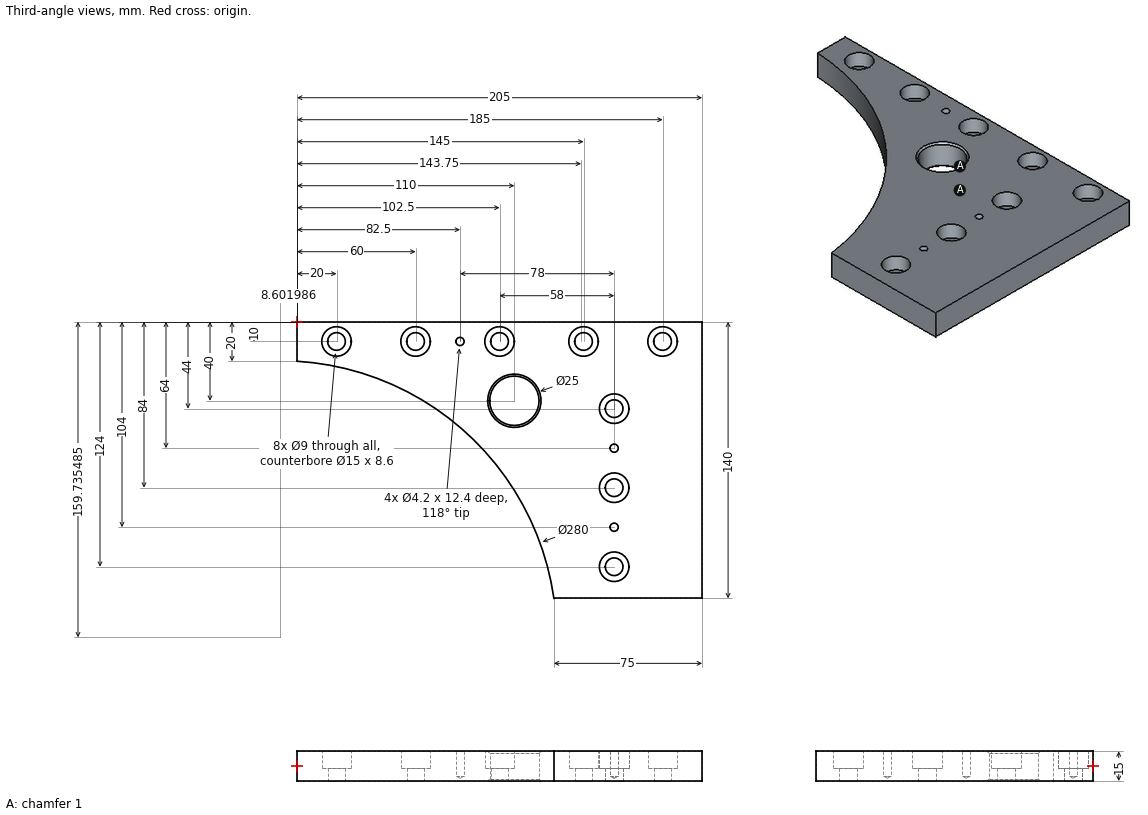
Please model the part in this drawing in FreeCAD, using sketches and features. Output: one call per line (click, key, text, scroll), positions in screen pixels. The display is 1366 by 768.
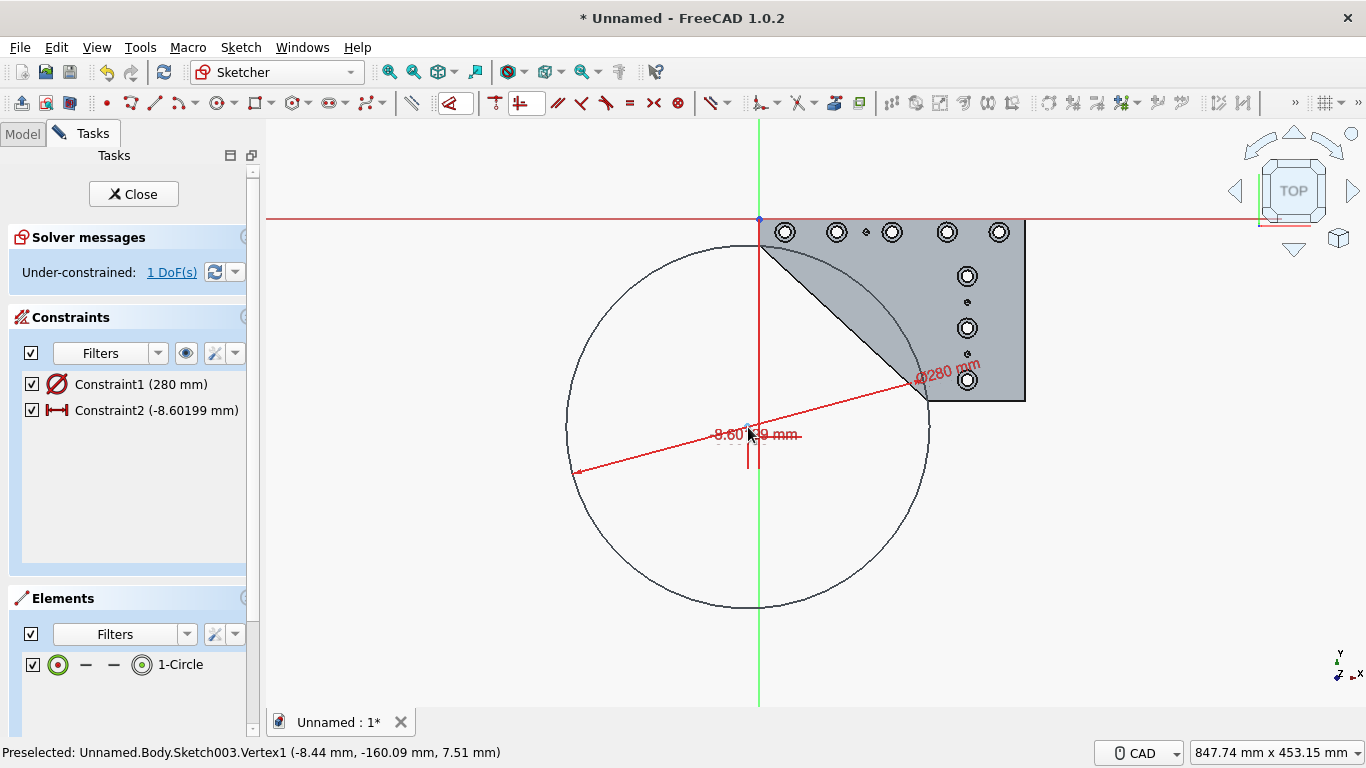
click(748, 427)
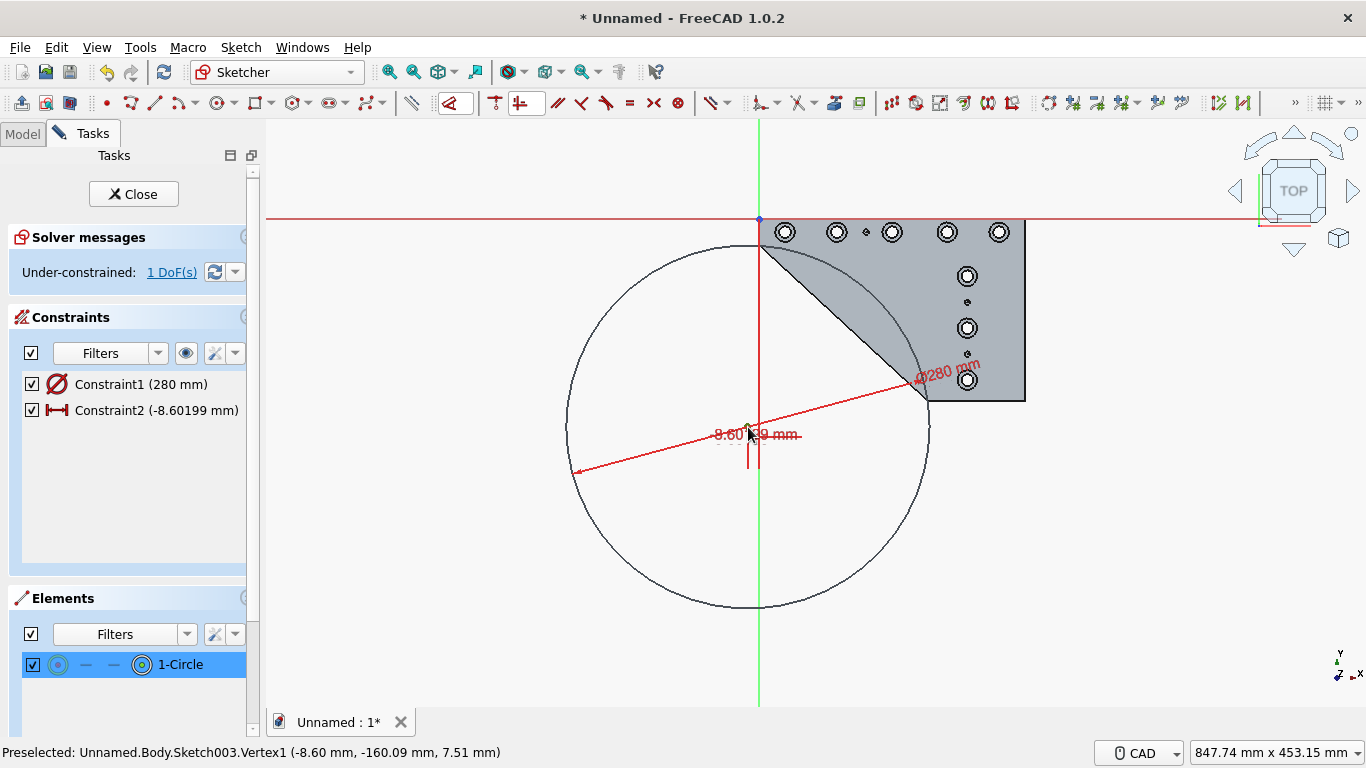
click(468, 104)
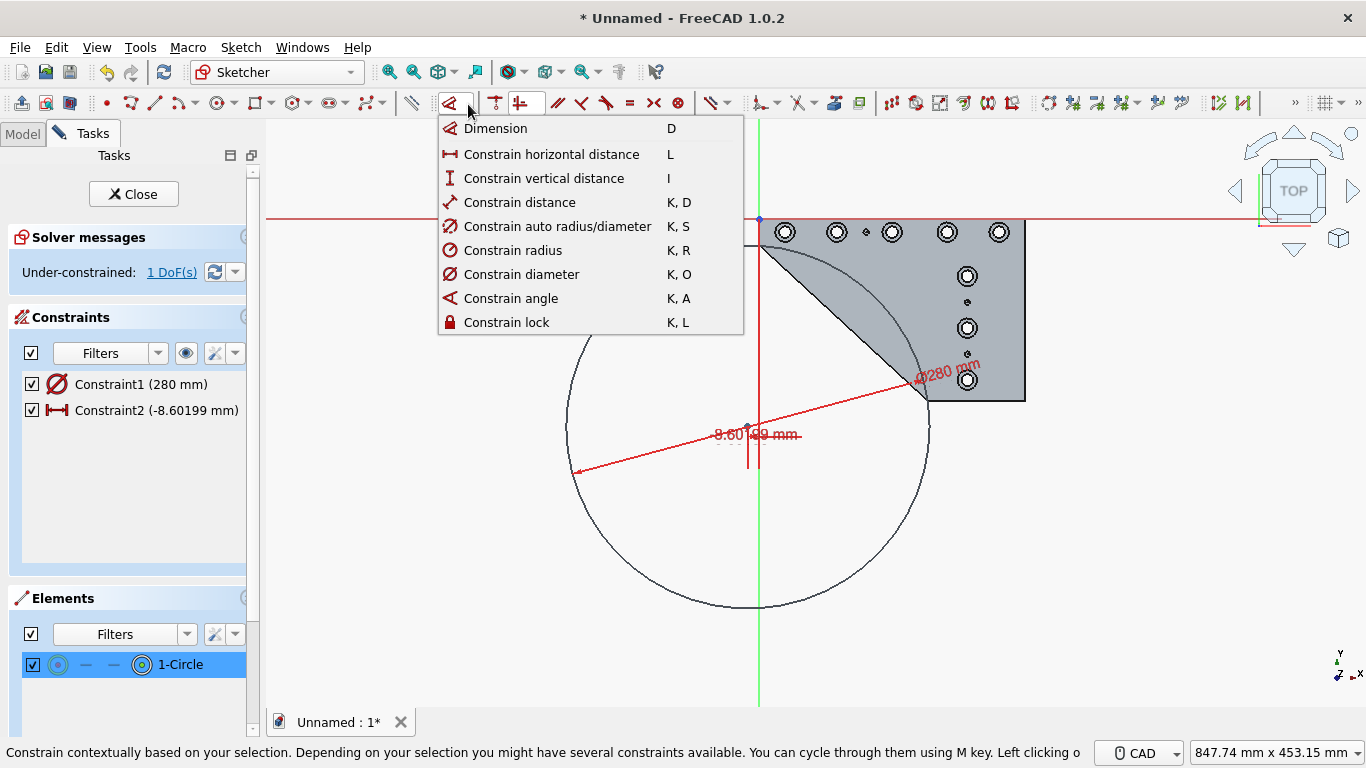
click(591, 178)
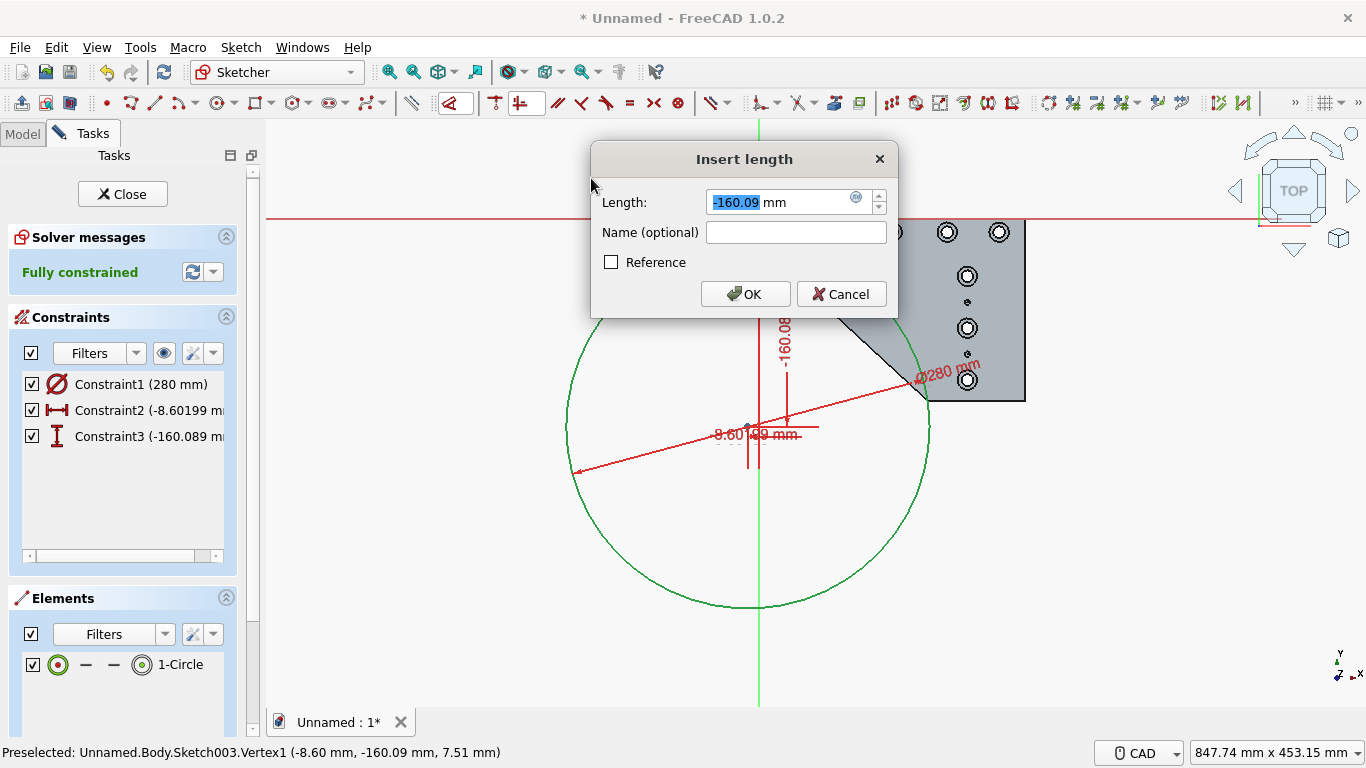
text(-159.735485)
key(Return)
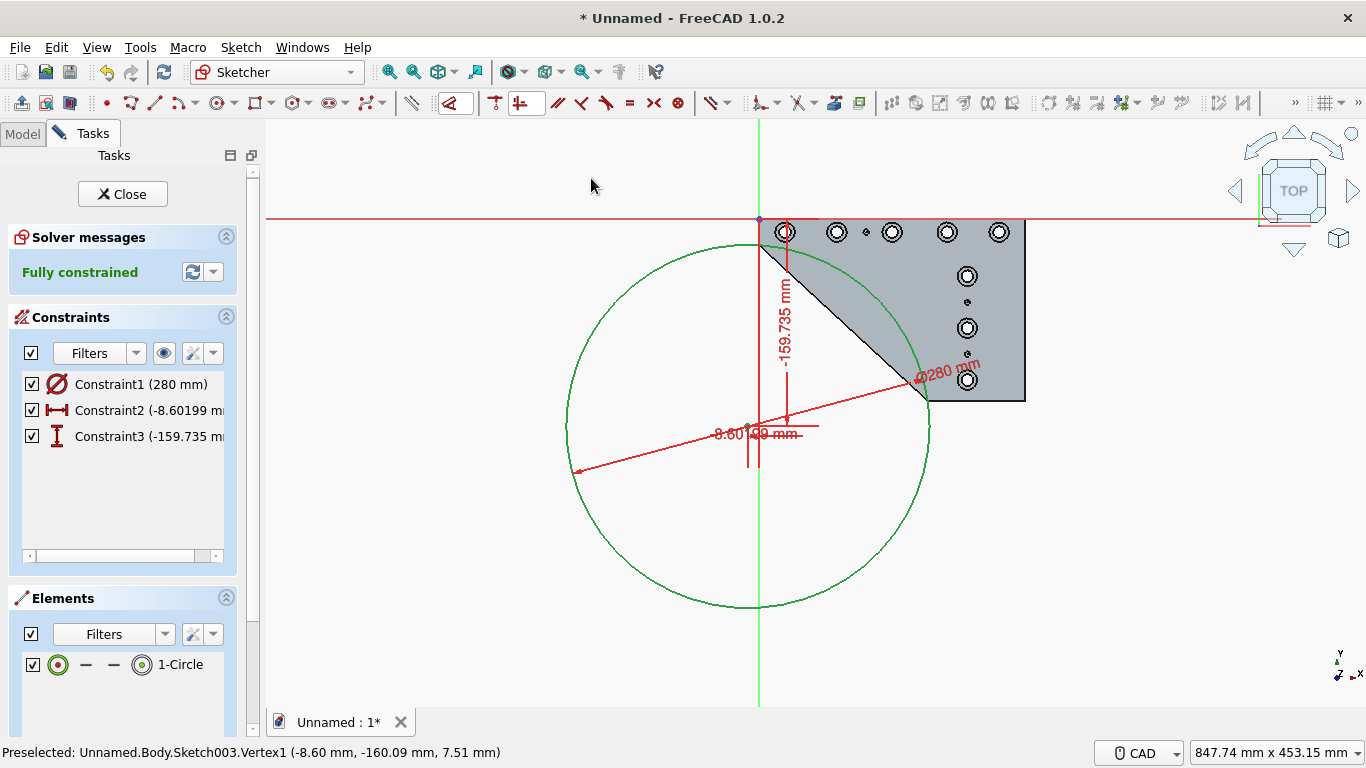
click(123, 194)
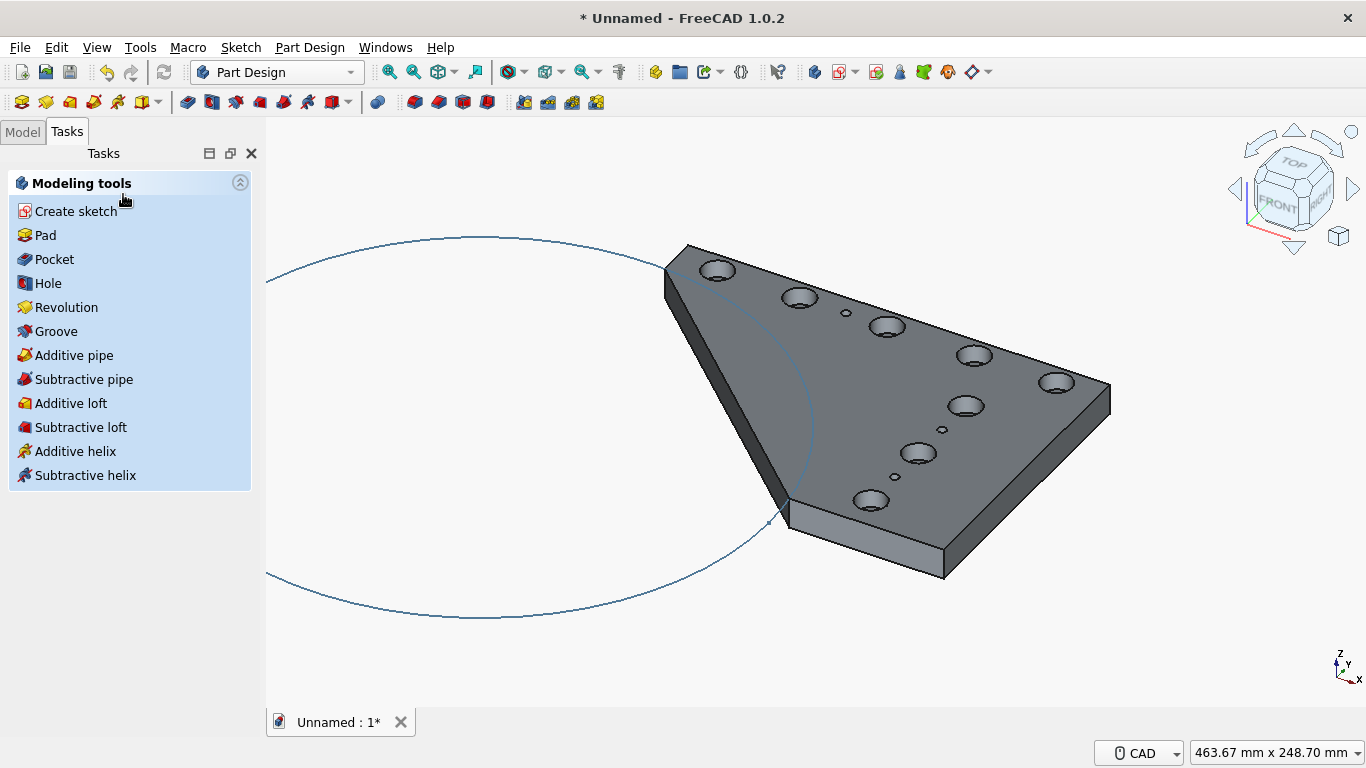
click(188, 102)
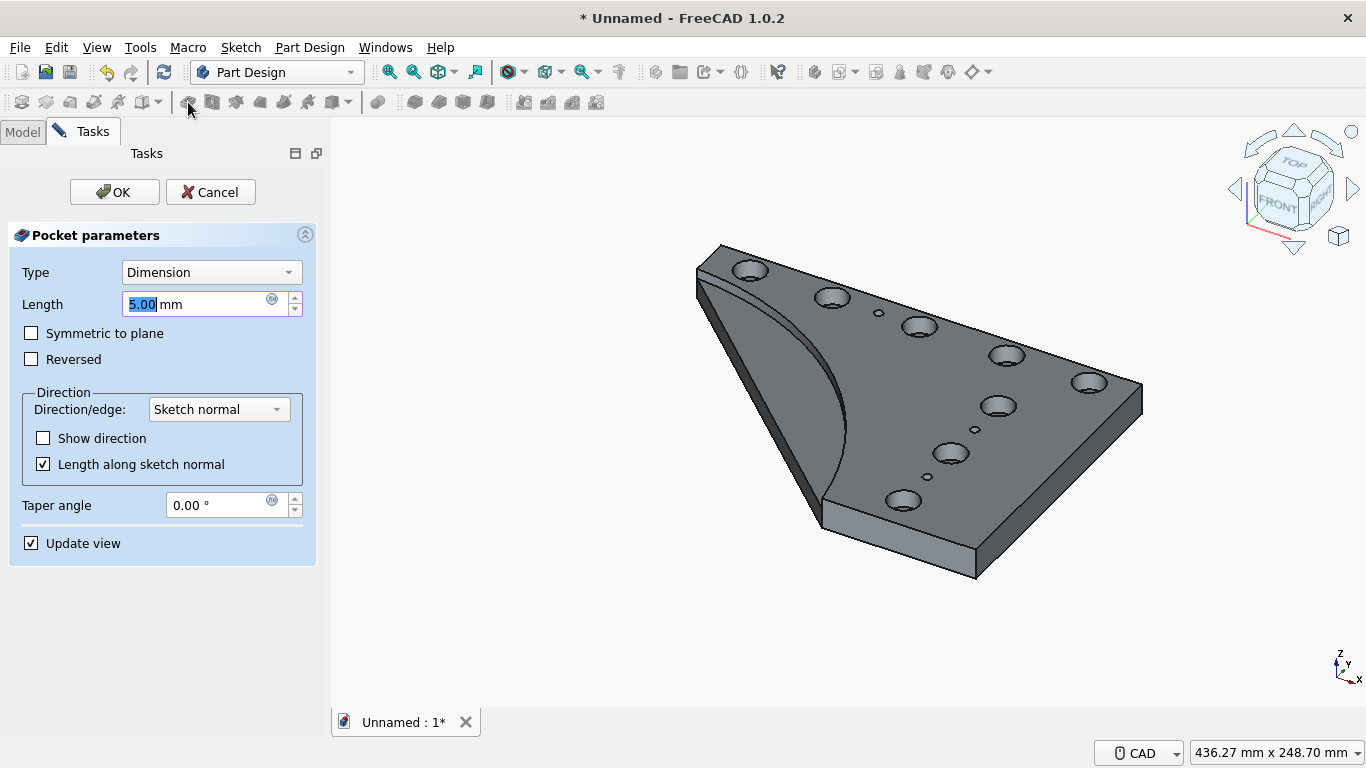
click(212, 272)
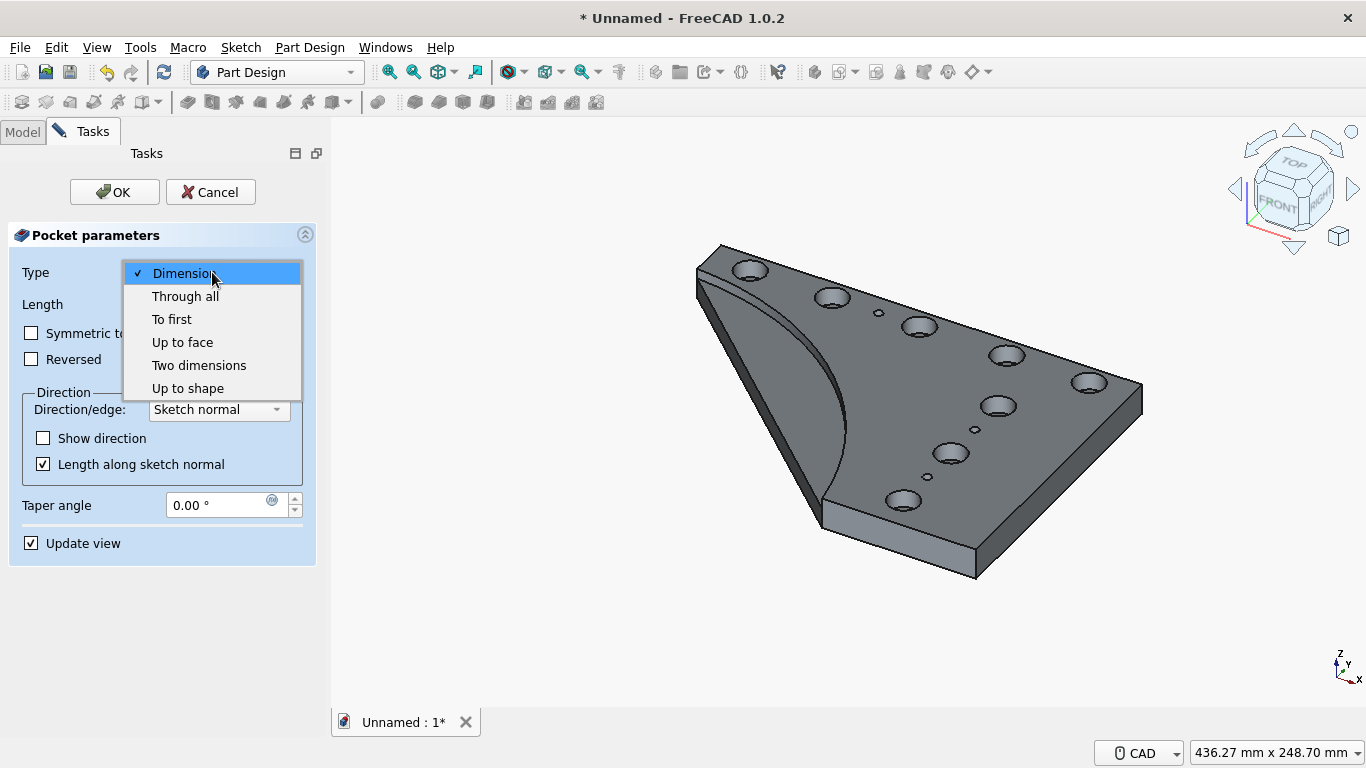
click(212, 296)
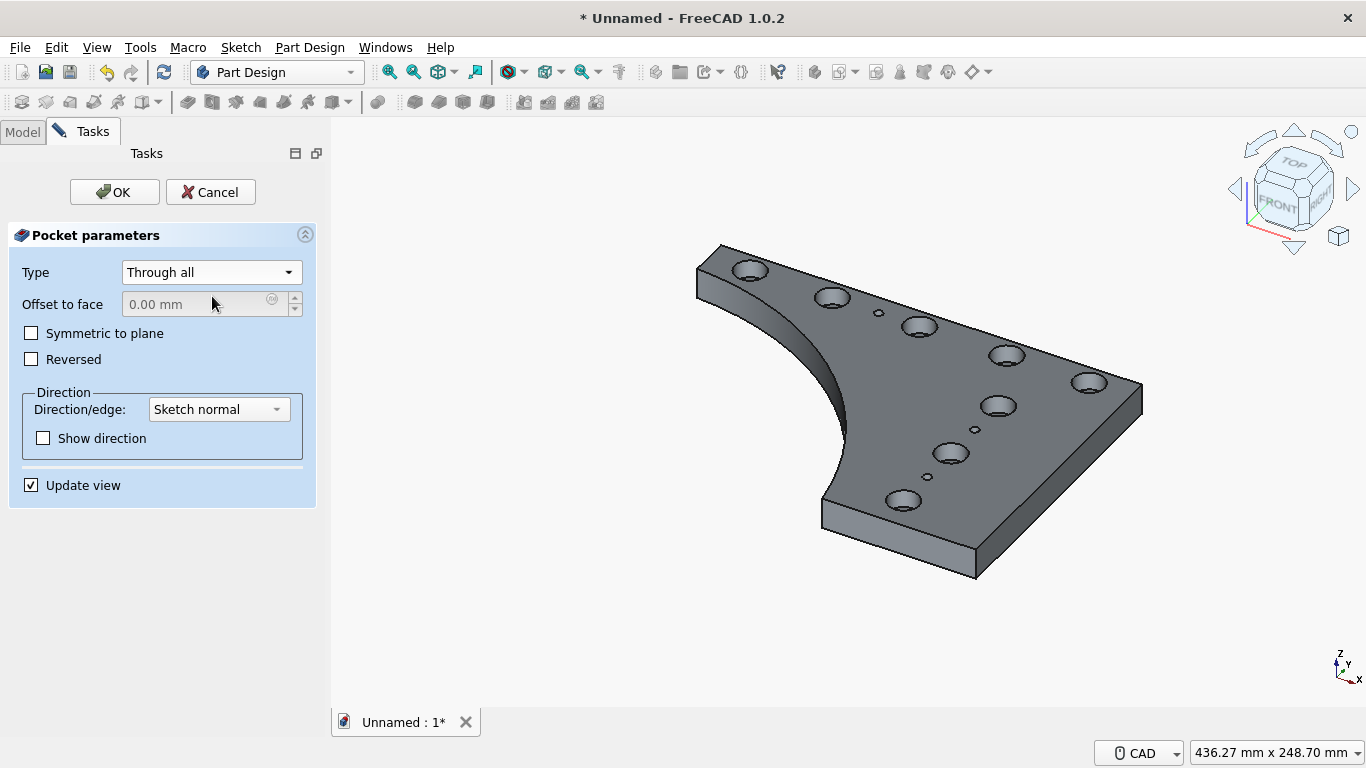
click(115, 192)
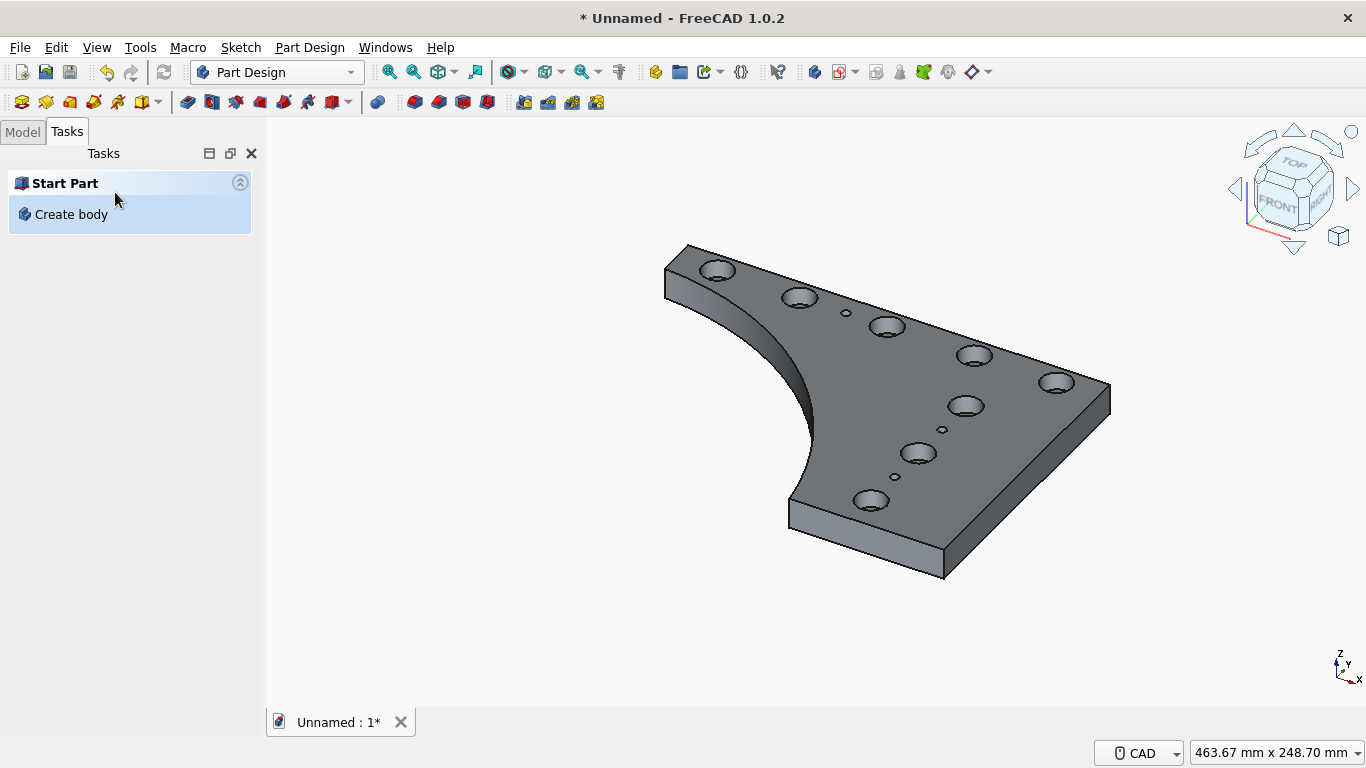
click(23, 131)